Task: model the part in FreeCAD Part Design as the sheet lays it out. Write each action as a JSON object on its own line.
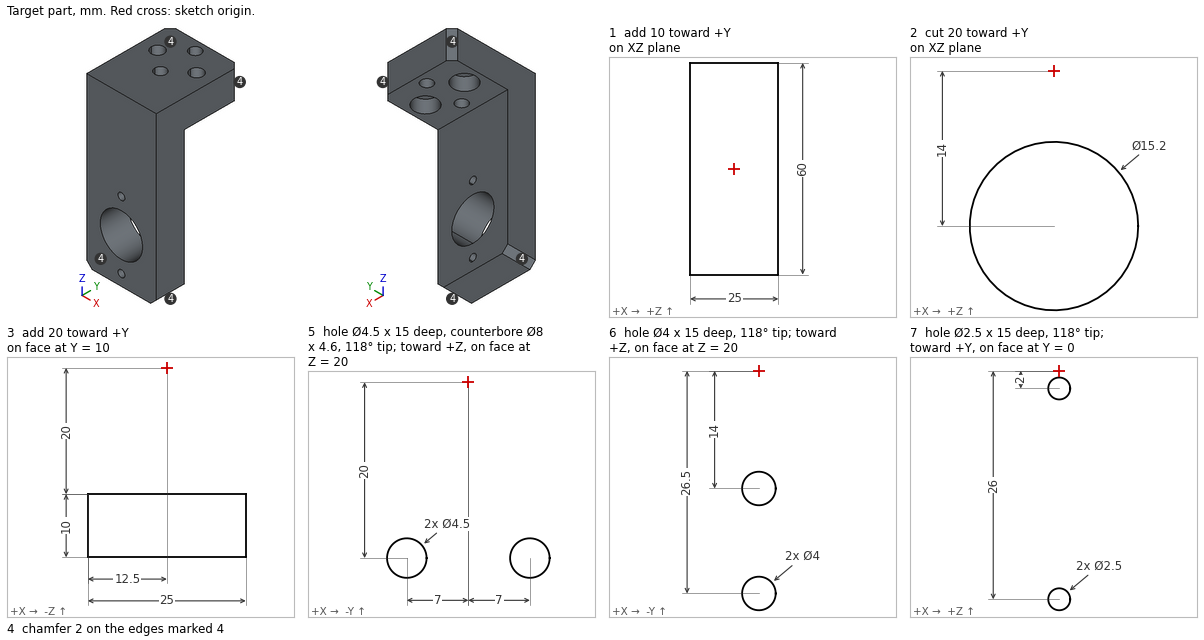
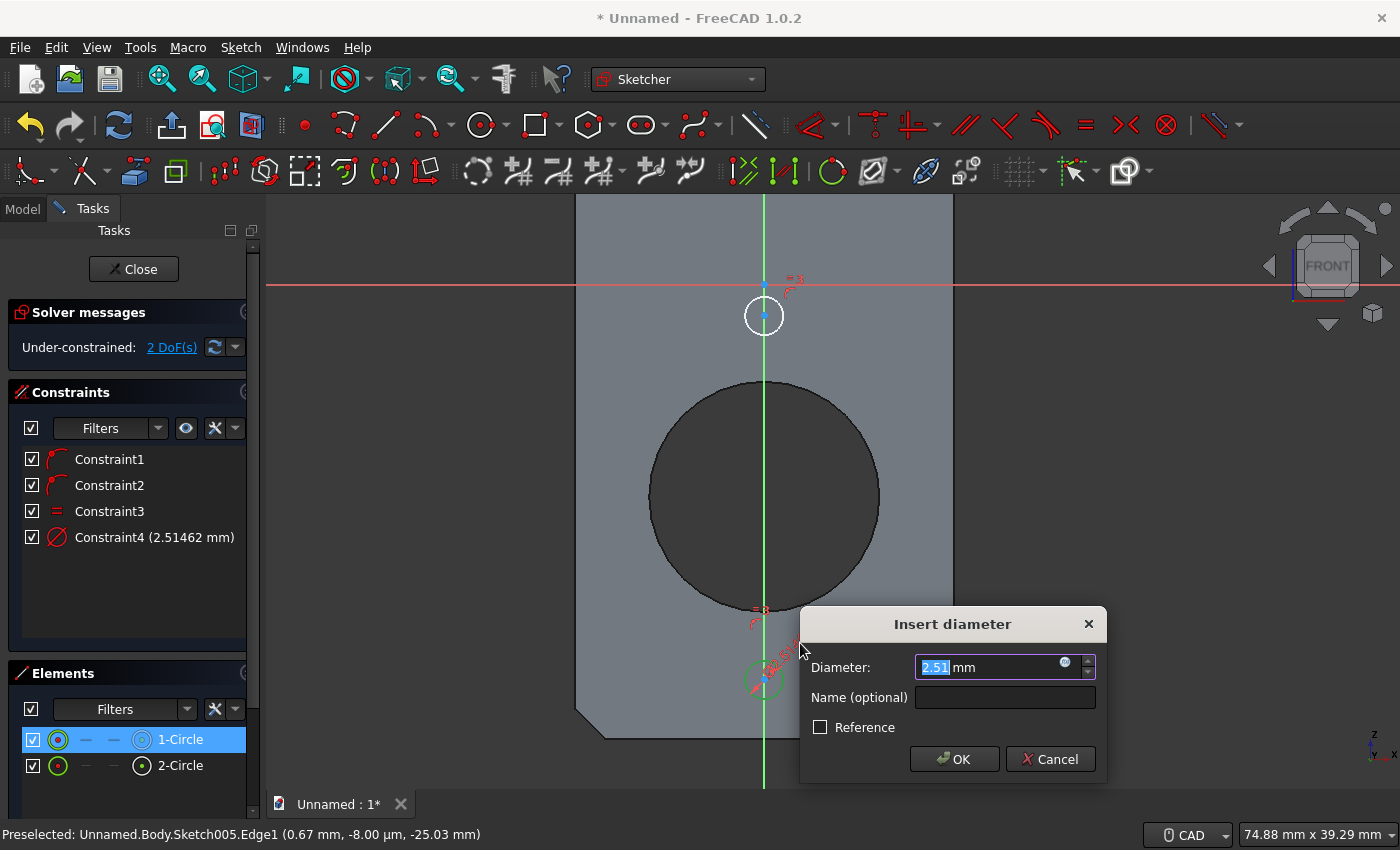
{"action": "type", "text": "2.5"}
{"action": "key", "text": "Return"}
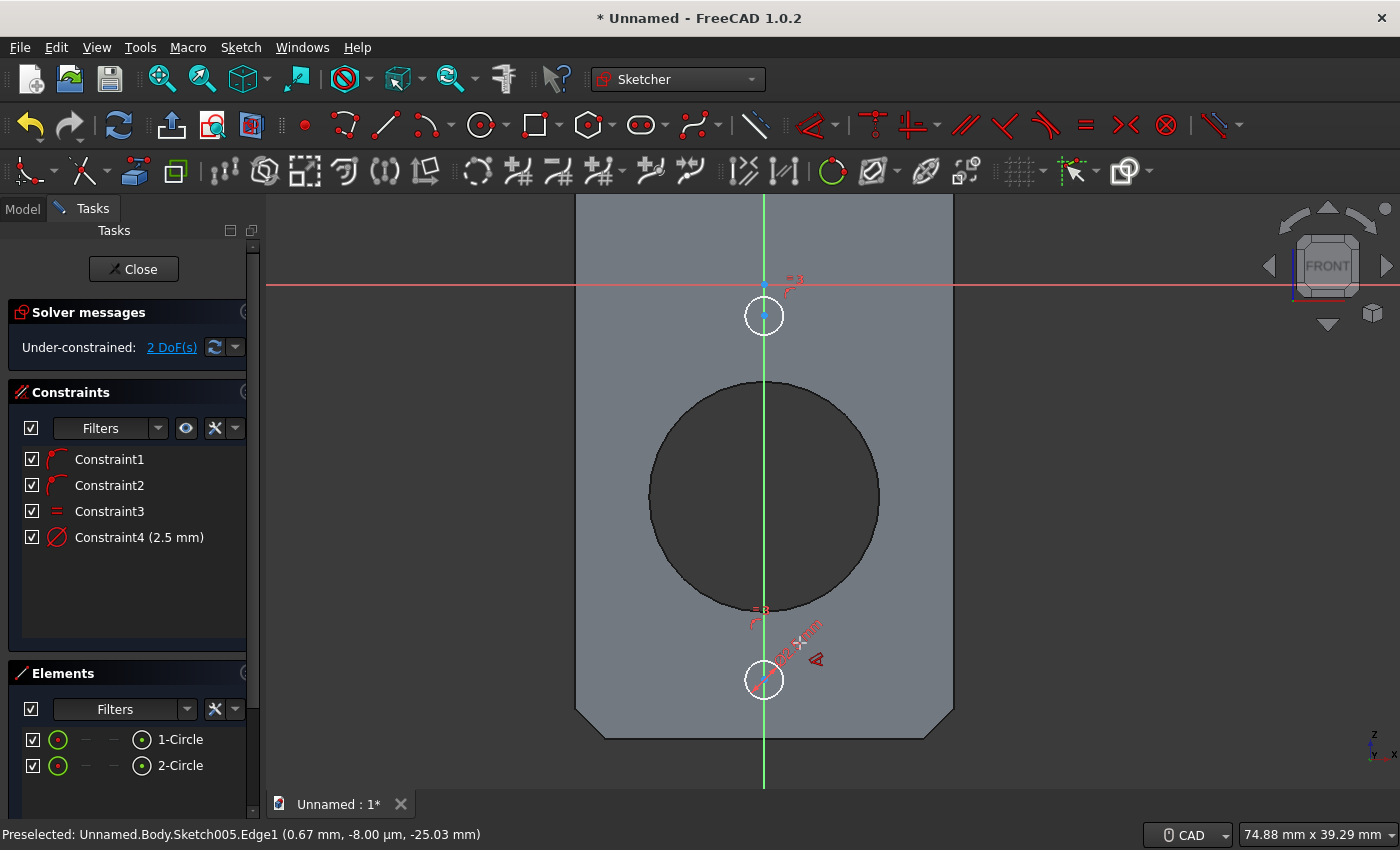
{"action": "scroll", "coordinate": [764, 316], "scroll_direction": "up", "scroll_amount": 2}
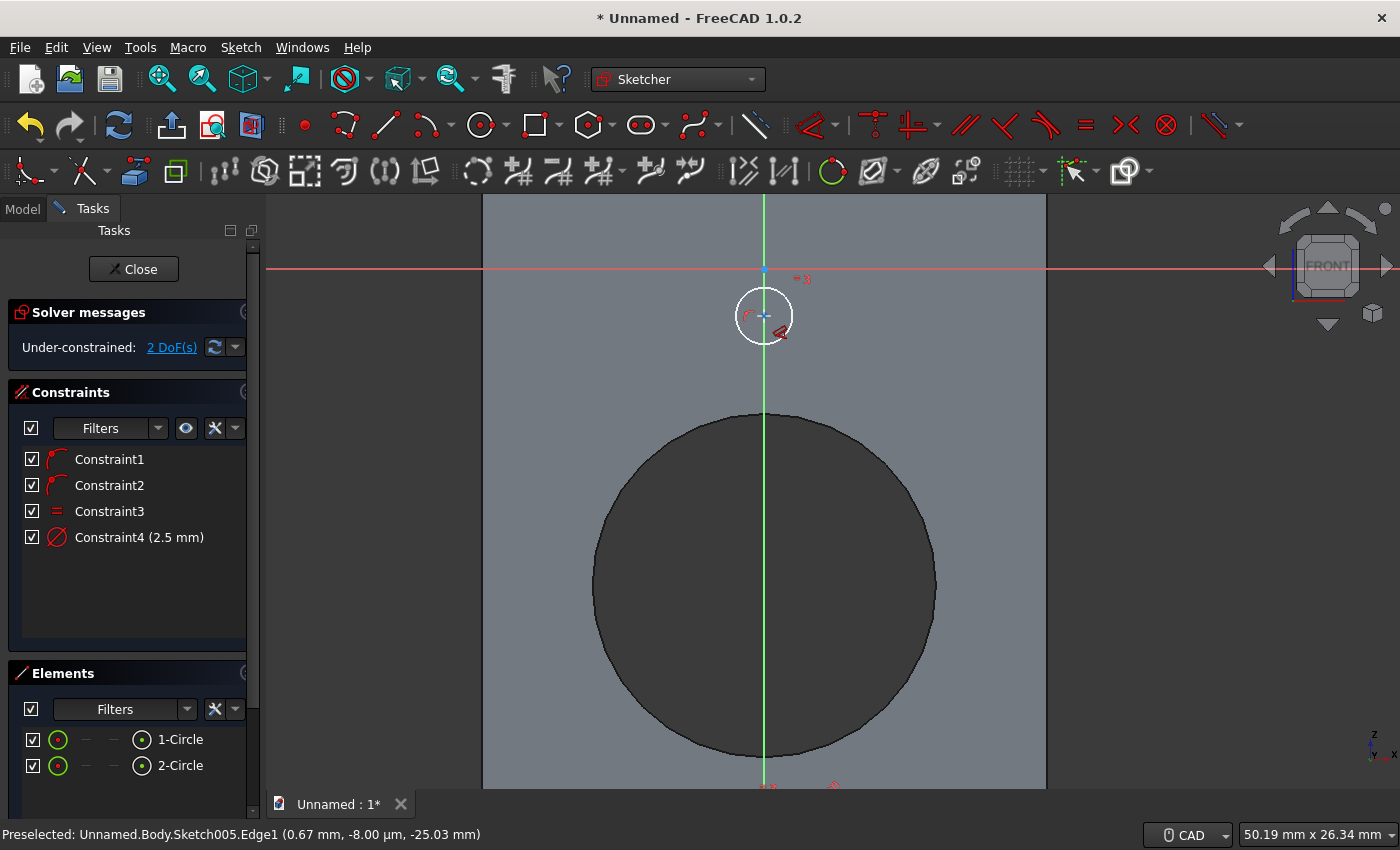
{"action": "left_click", "coordinate": [764, 316]}
{"action": "left_click", "coordinate": [822, 293]}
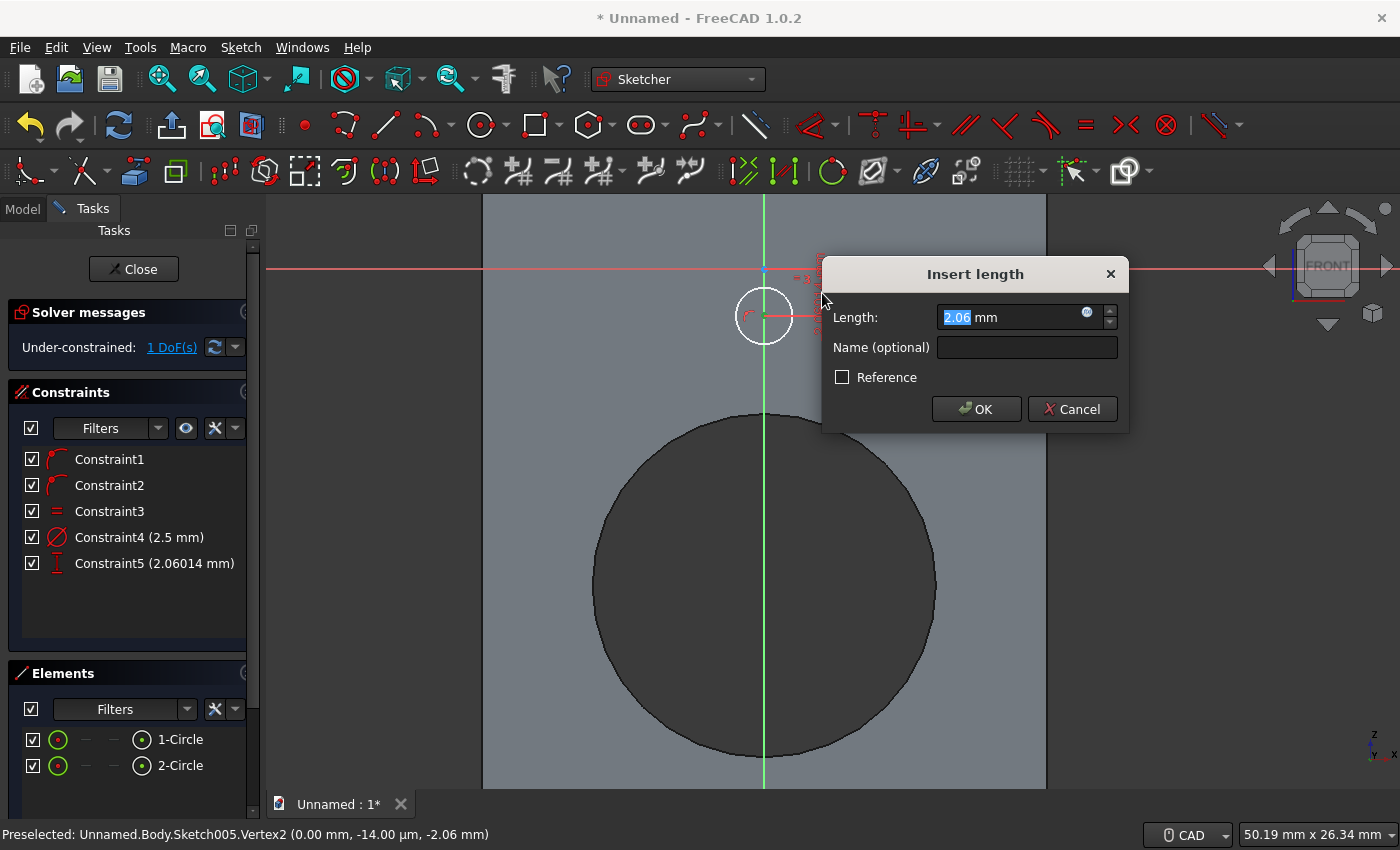
{"action": "type", "text": "2"}
{"action": "key", "text": "Return"}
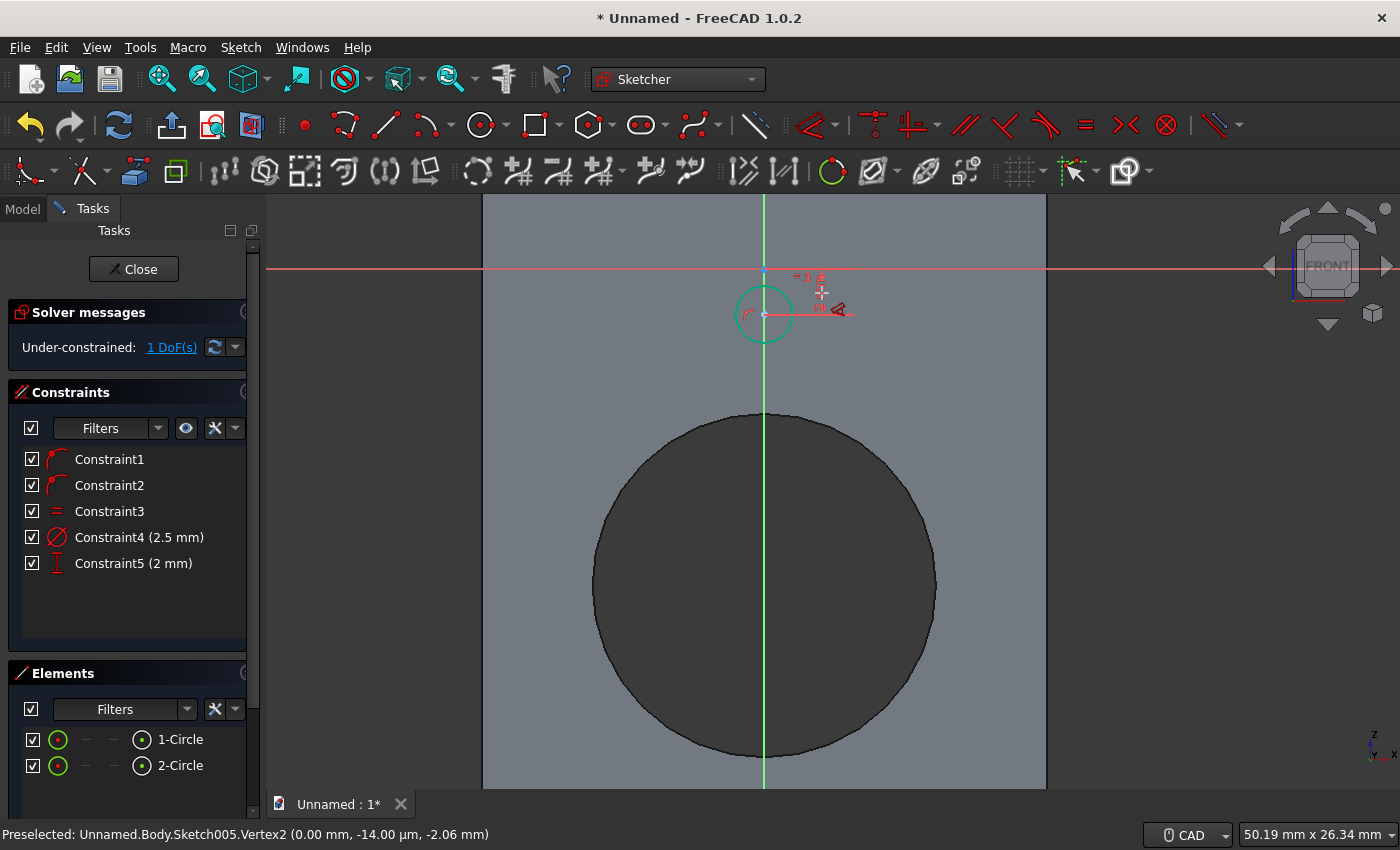
{"action": "scroll", "coordinate": [765, 317], "scroll_direction": "down", "scroll_amount": 2}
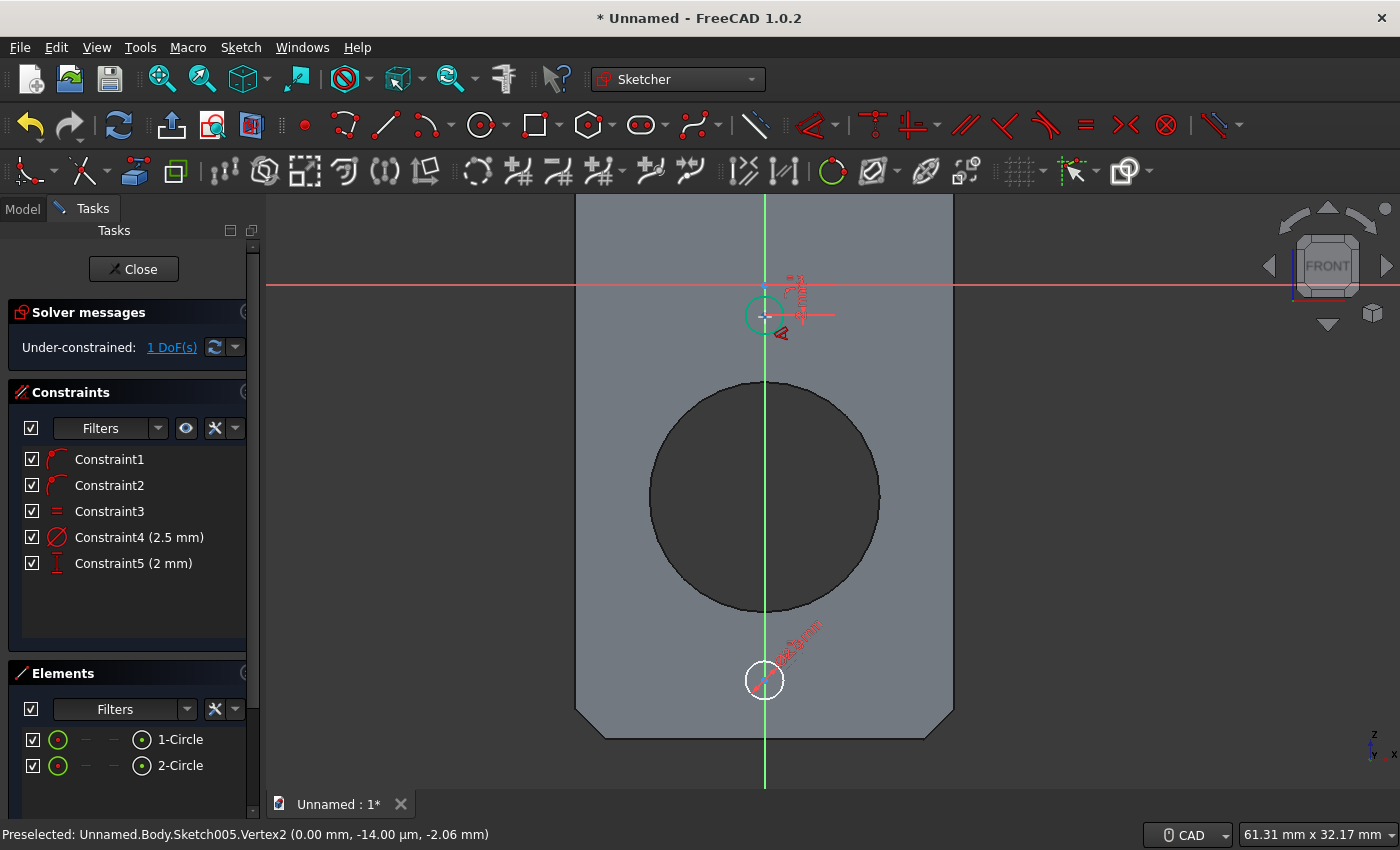
{"action": "left_click", "coordinate": [765, 680]}
{"action": "left_click", "coordinate": [799, 483]}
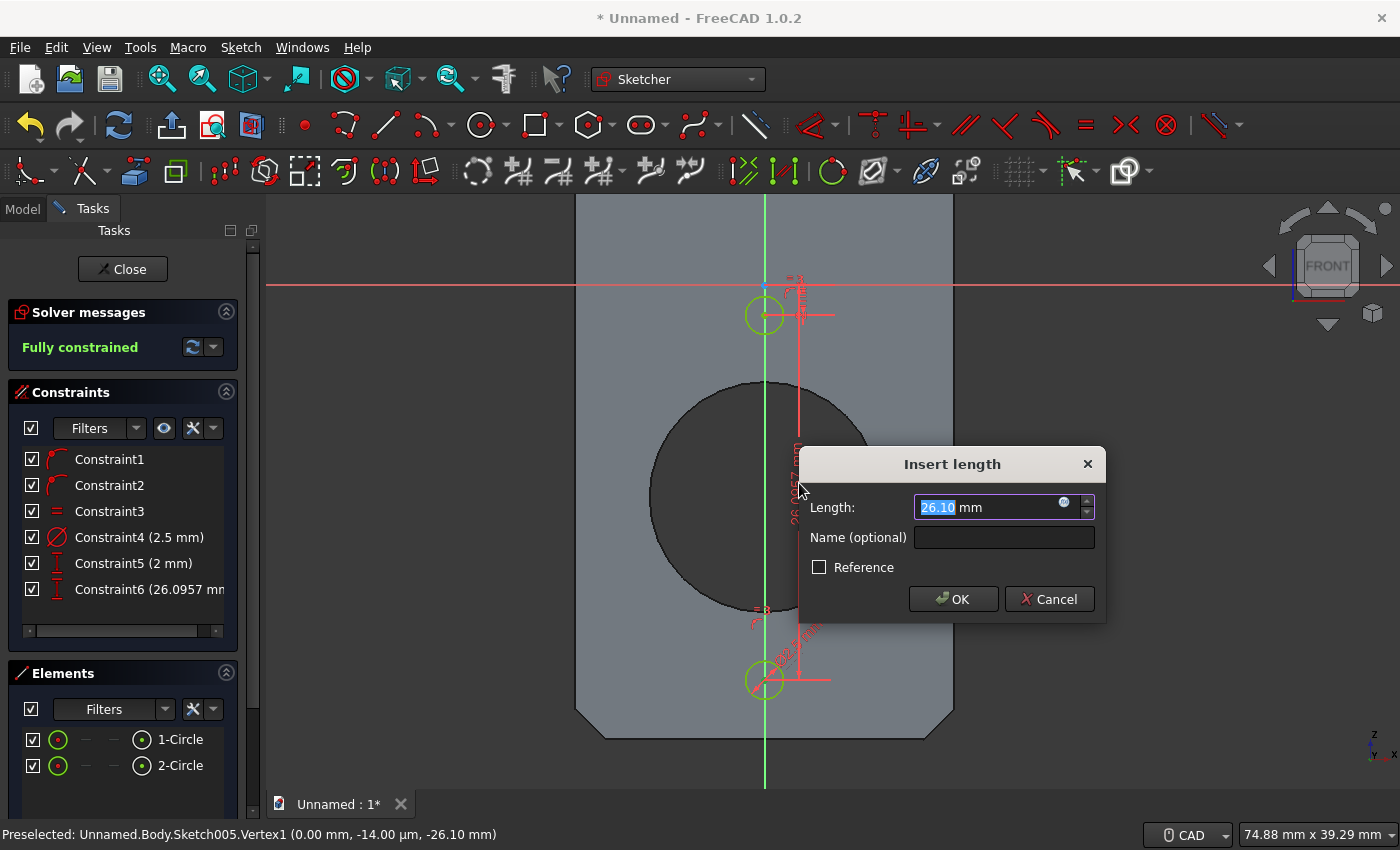
{"action": "type", "text": "26"}
{"action": "key", "text": "Return"}
{"action": "key", "text": "Escape"}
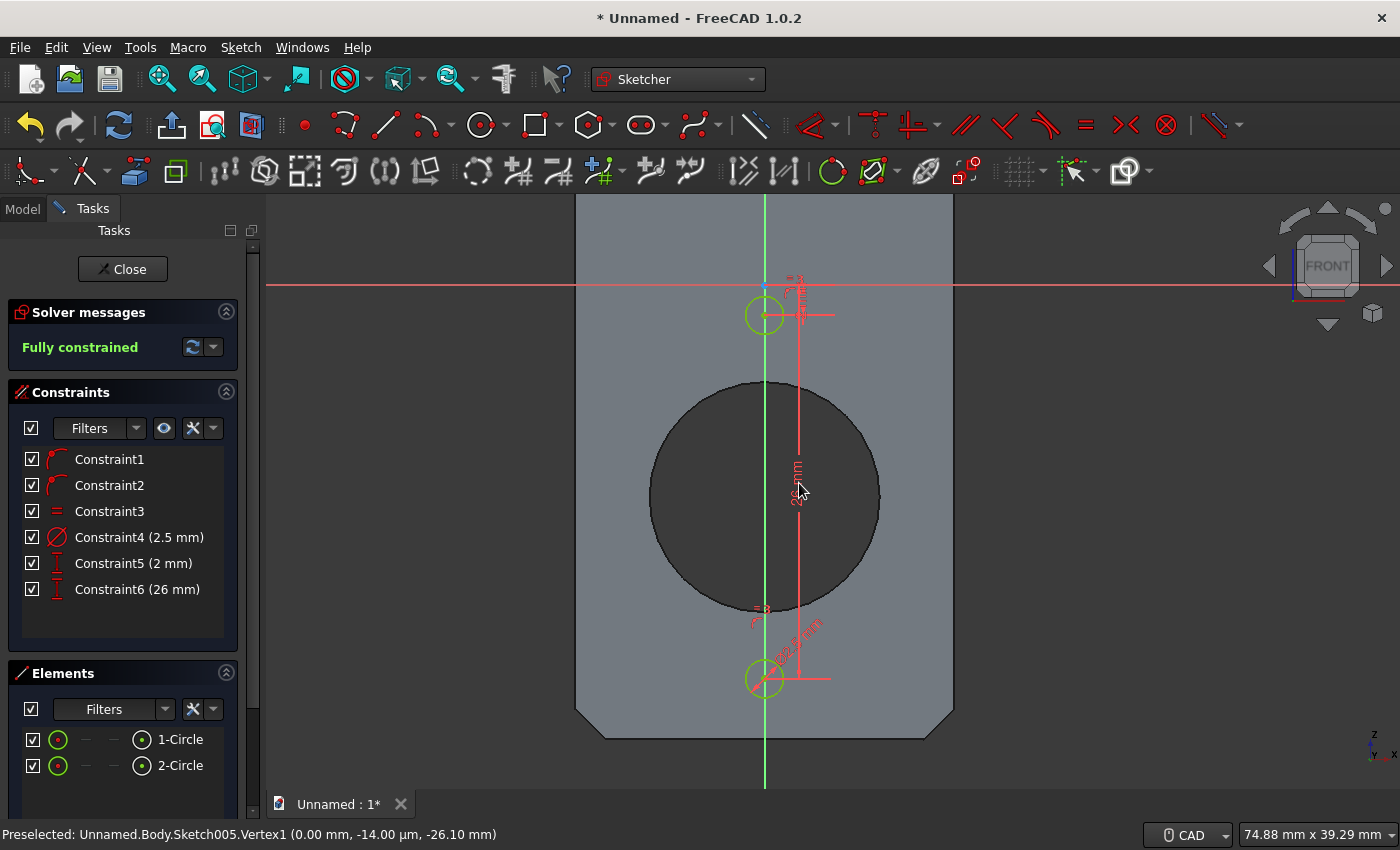
{"action": "left_click", "coordinate": [123, 269]}